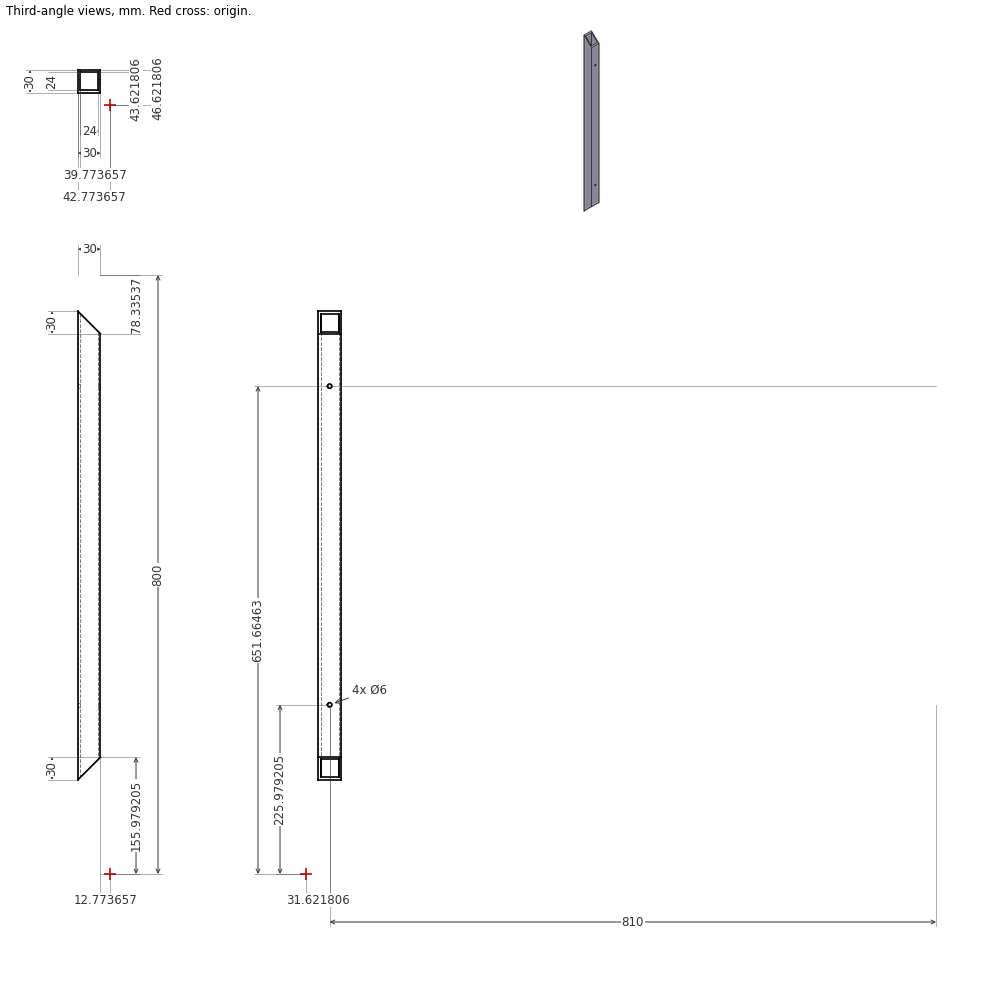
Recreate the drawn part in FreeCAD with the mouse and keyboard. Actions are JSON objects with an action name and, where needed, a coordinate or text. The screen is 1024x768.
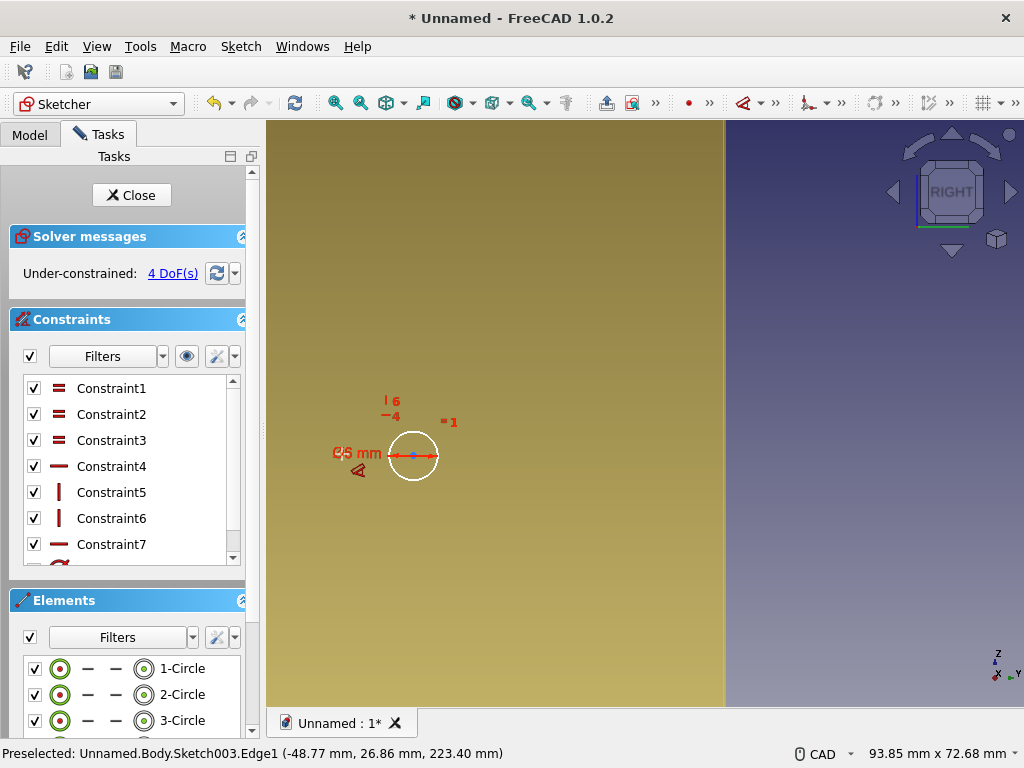
{"action": "scroll", "coordinate": [383, 465], "scroll_direction": "down", "scroll_amount": 14}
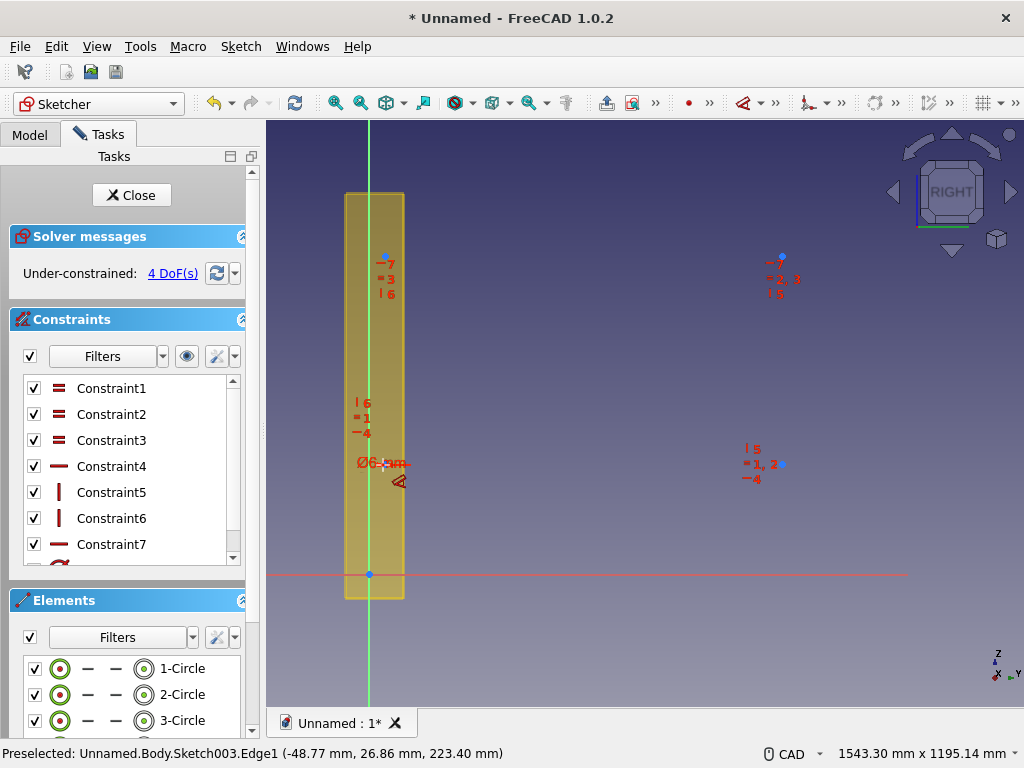
{"action": "left_click", "coordinate": [385, 465]}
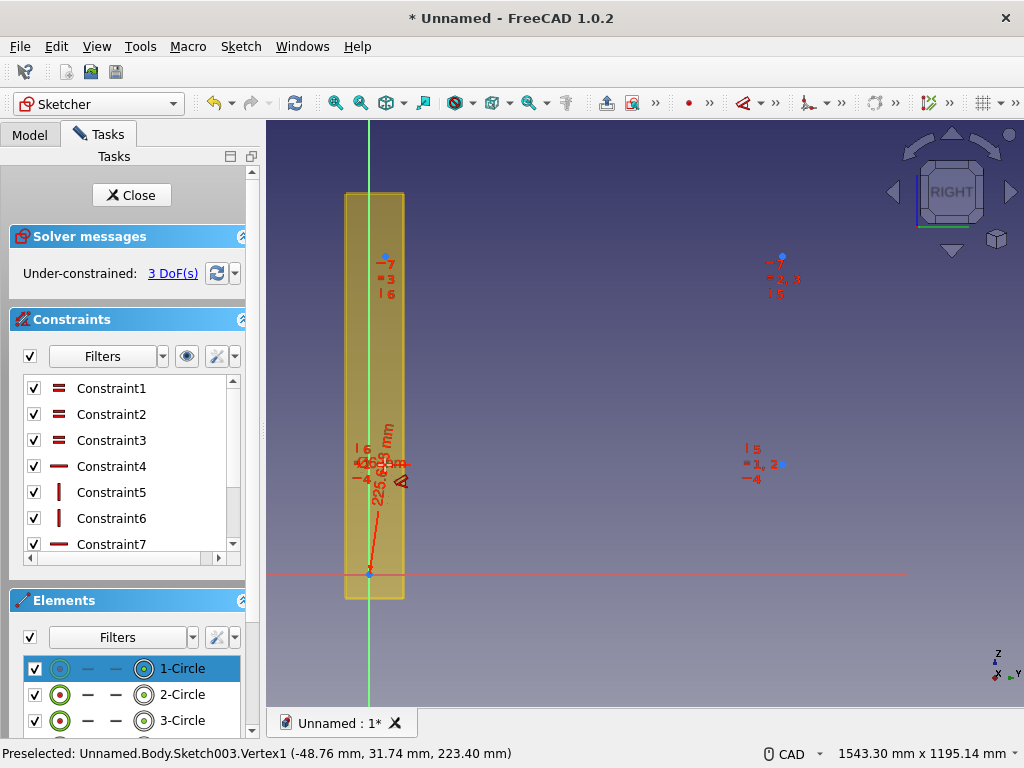
{"action": "left_click", "coordinate": [783, 465]}
{"action": "left_click", "coordinate": [584, 499]}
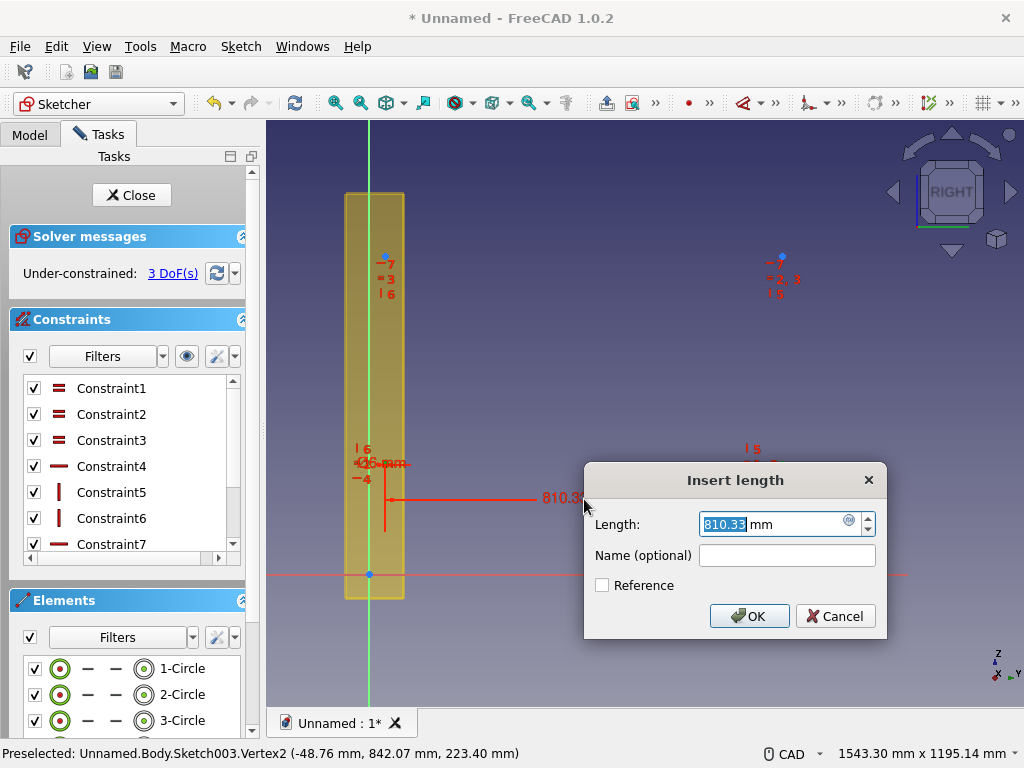
{"action": "type", "text": "810"}
{"action": "key", "text": "Return"}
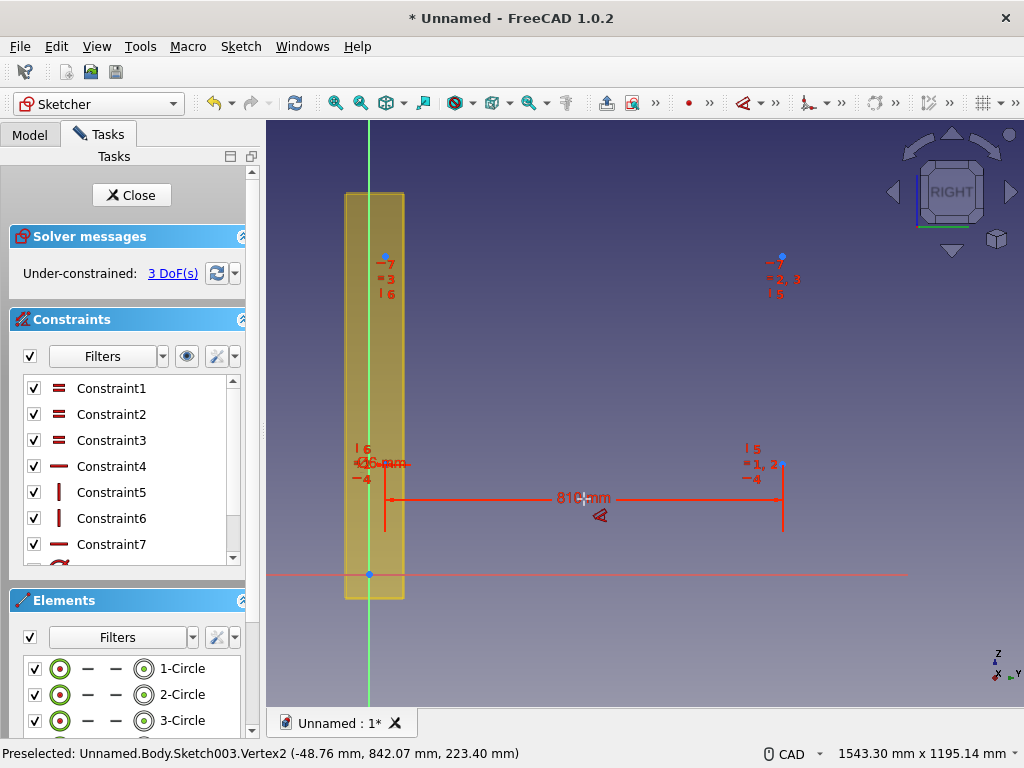
{"action": "scroll", "coordinate": [385, 465], "scroll_direction": "up", "scroll_amount": 5}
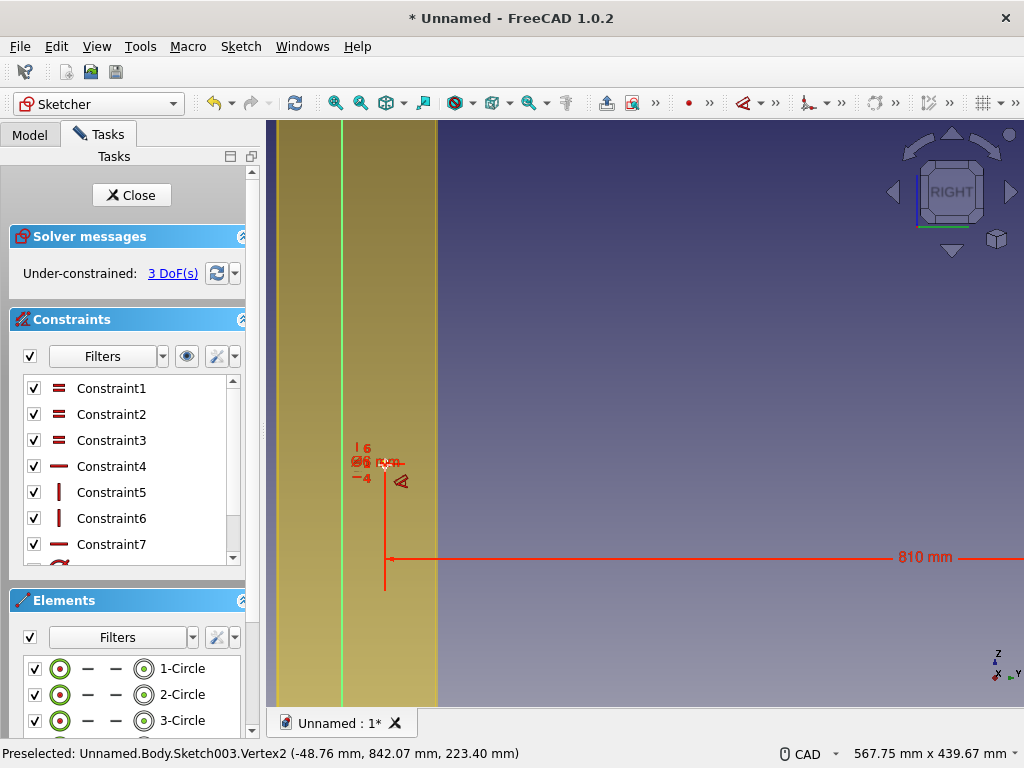
{"action": "left_click", "coordinate": [385, 464]}
{"action": "left_click", "coordinate": [364, 430]}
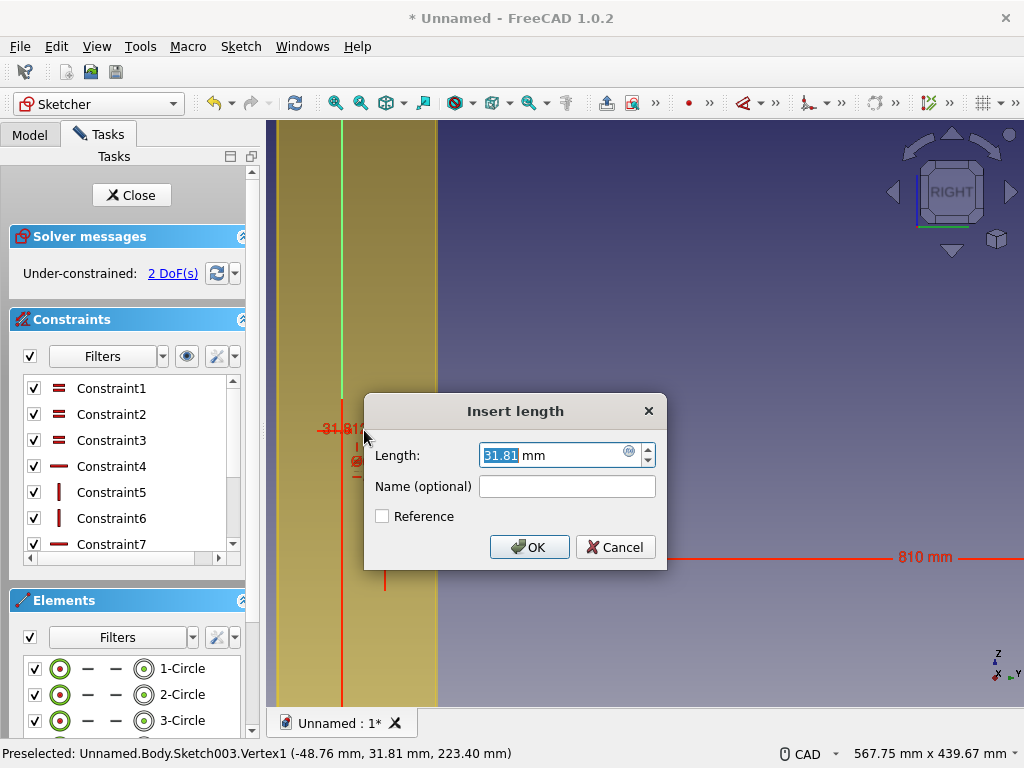
{"action": "type", "text": "31.621806"}
{"action": "key", "text": "Return"}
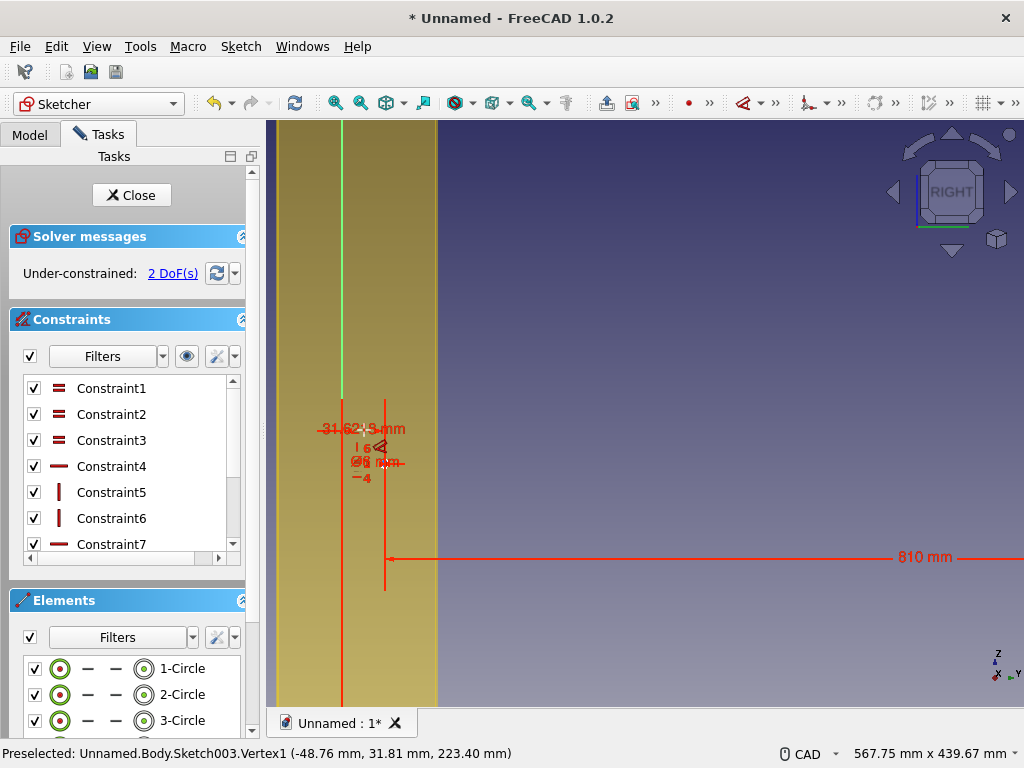
{"action": "scroll", "coordinate": [385, 465], "scroll_direction": "down", "scroll_amount": 5}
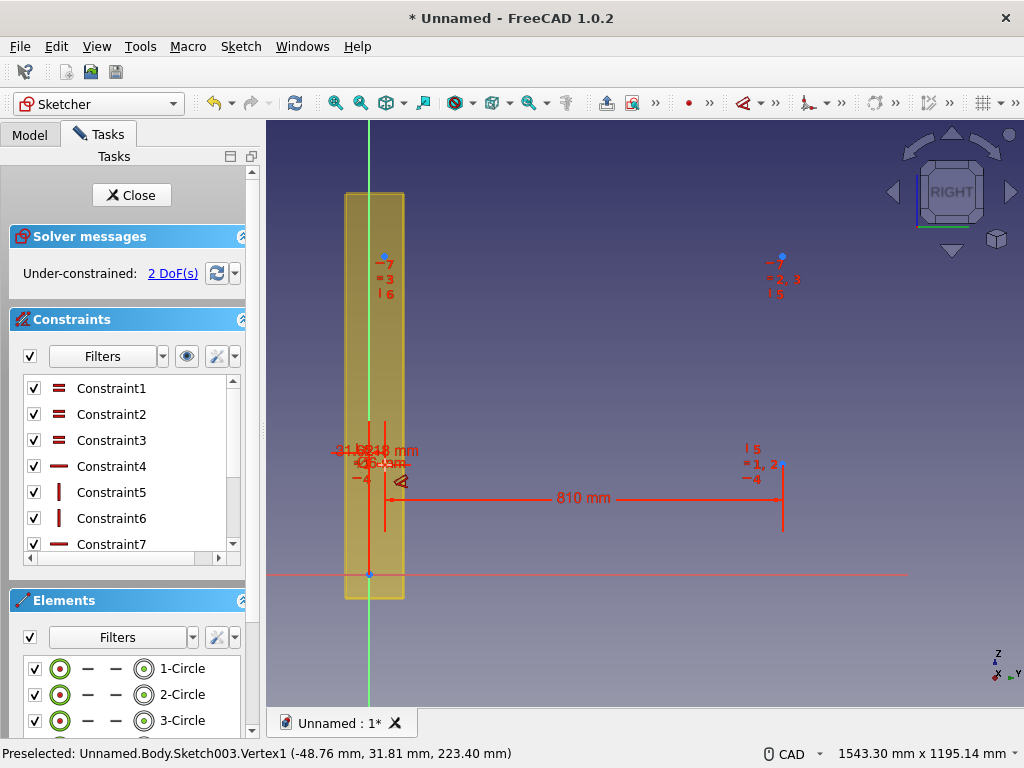
{"action": "left_click", "coordinate": [783, 256]}
{"action": "left_click", "coordinate": [335, 415]}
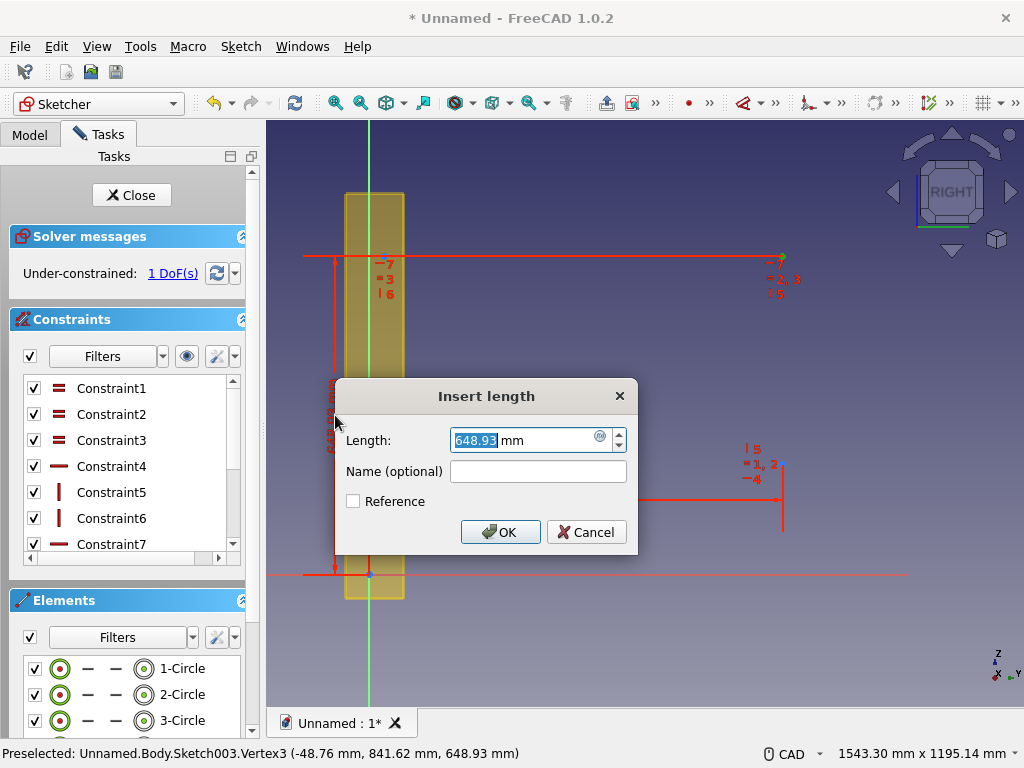
{"action": "type", "text": "651.66463"}
{"action": "key", "text": "Return"}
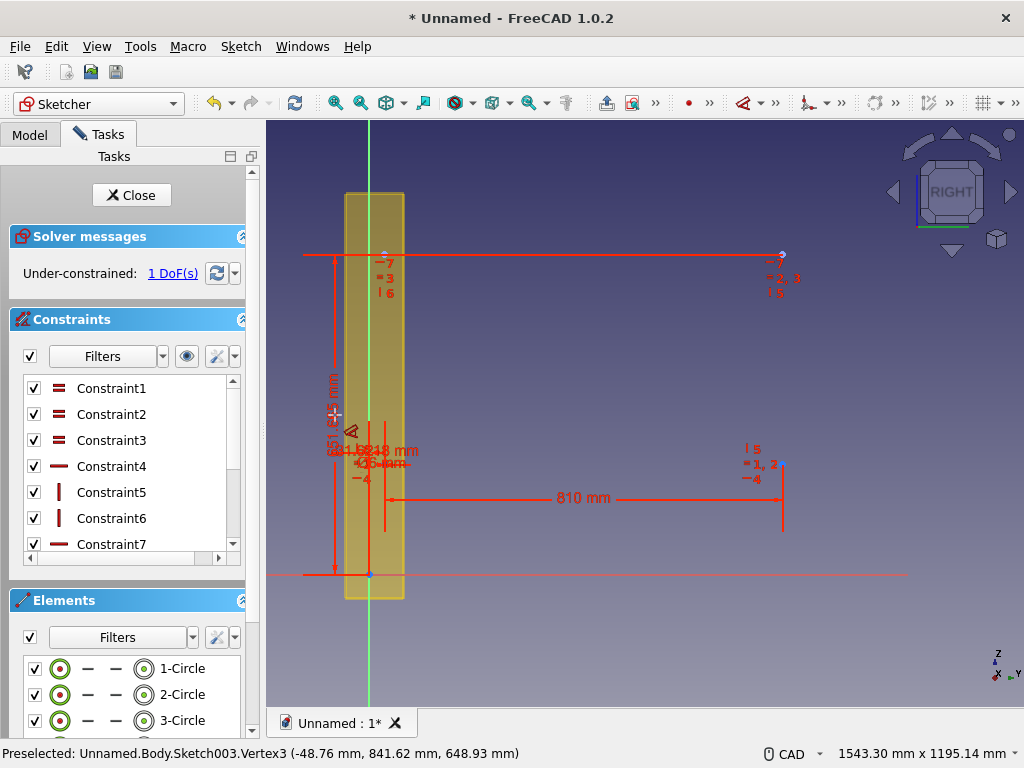
{"action": "left_click", "coordinate": [385, 465]}
{"action": "left_click", "coordinate": [335, 520]}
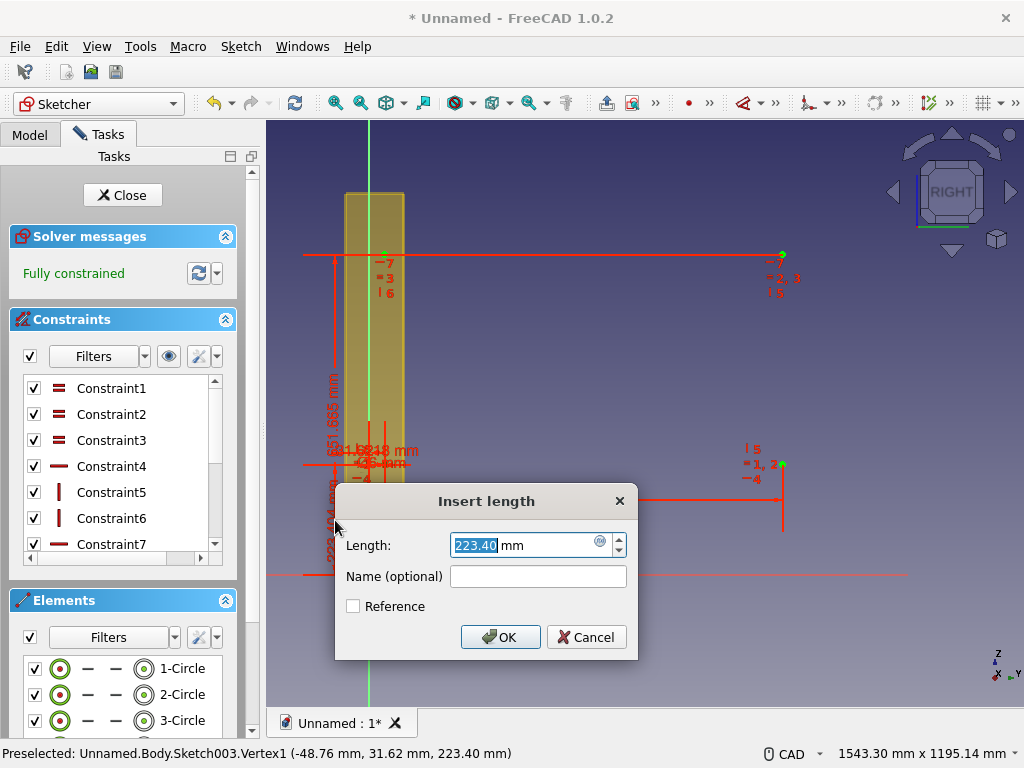
{"action": "type", "text": "225.979205"}
{"action": "key", "text": "Return"}
{"action": "key", "text": "Escape"}